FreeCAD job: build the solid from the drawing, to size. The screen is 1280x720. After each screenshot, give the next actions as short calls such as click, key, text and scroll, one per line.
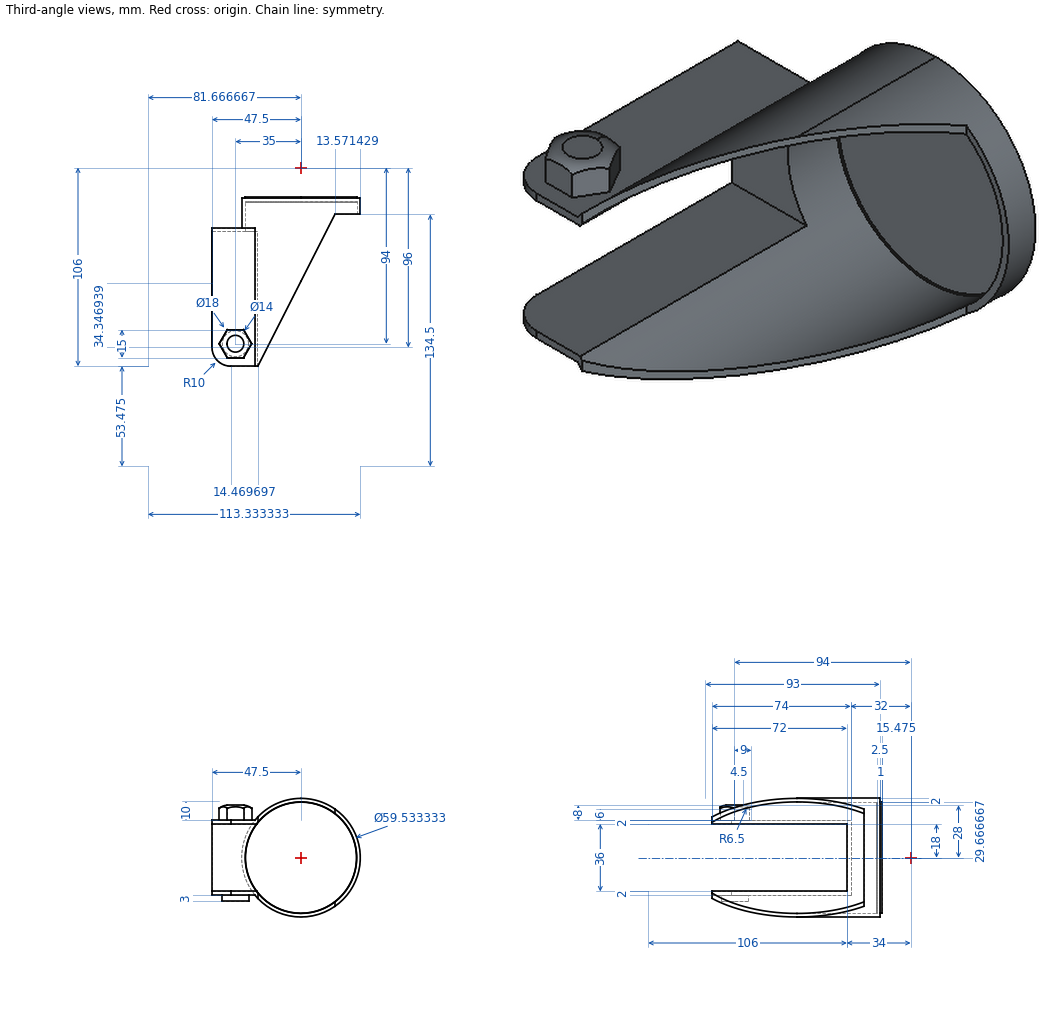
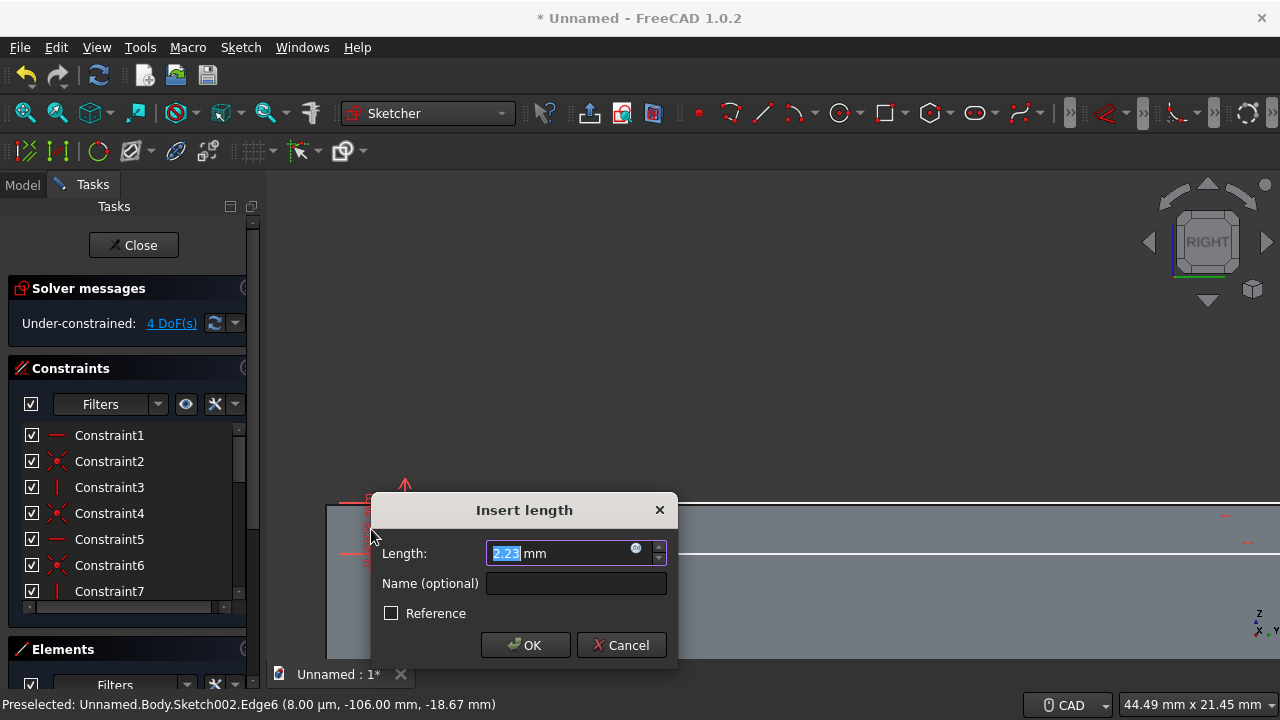
text(2)
key(Return)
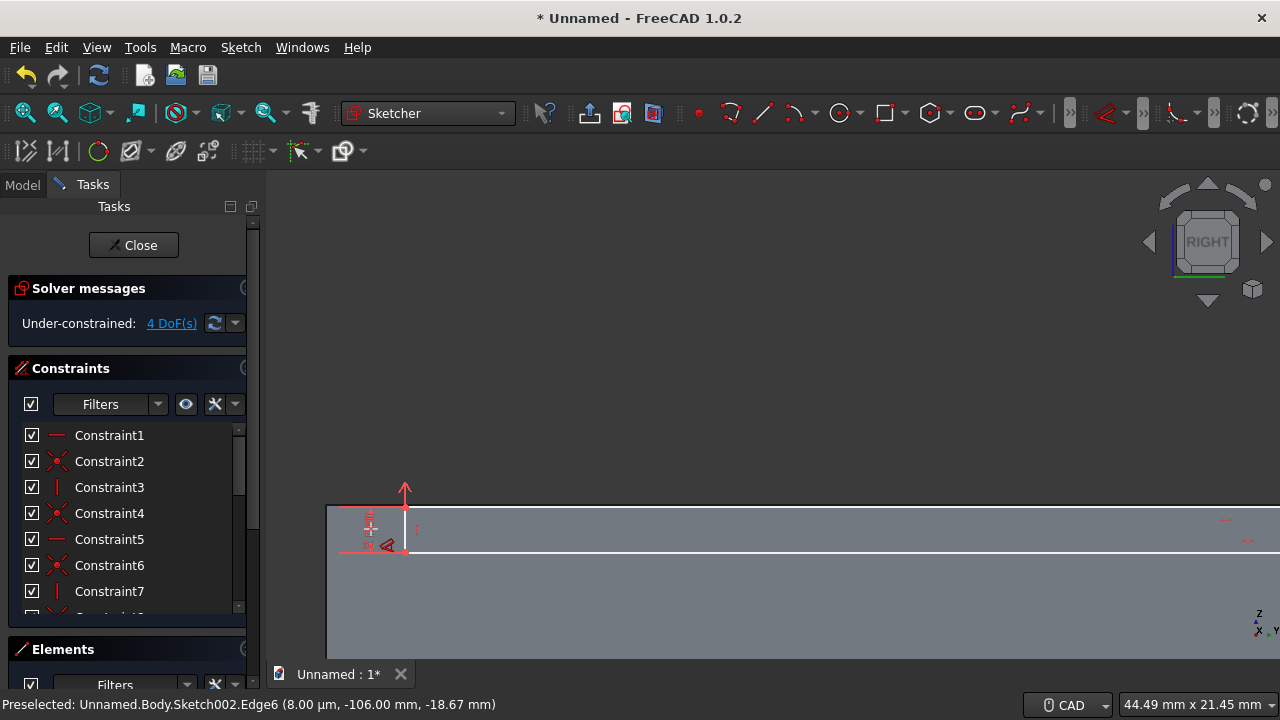
scroll(407, 519, down, 7)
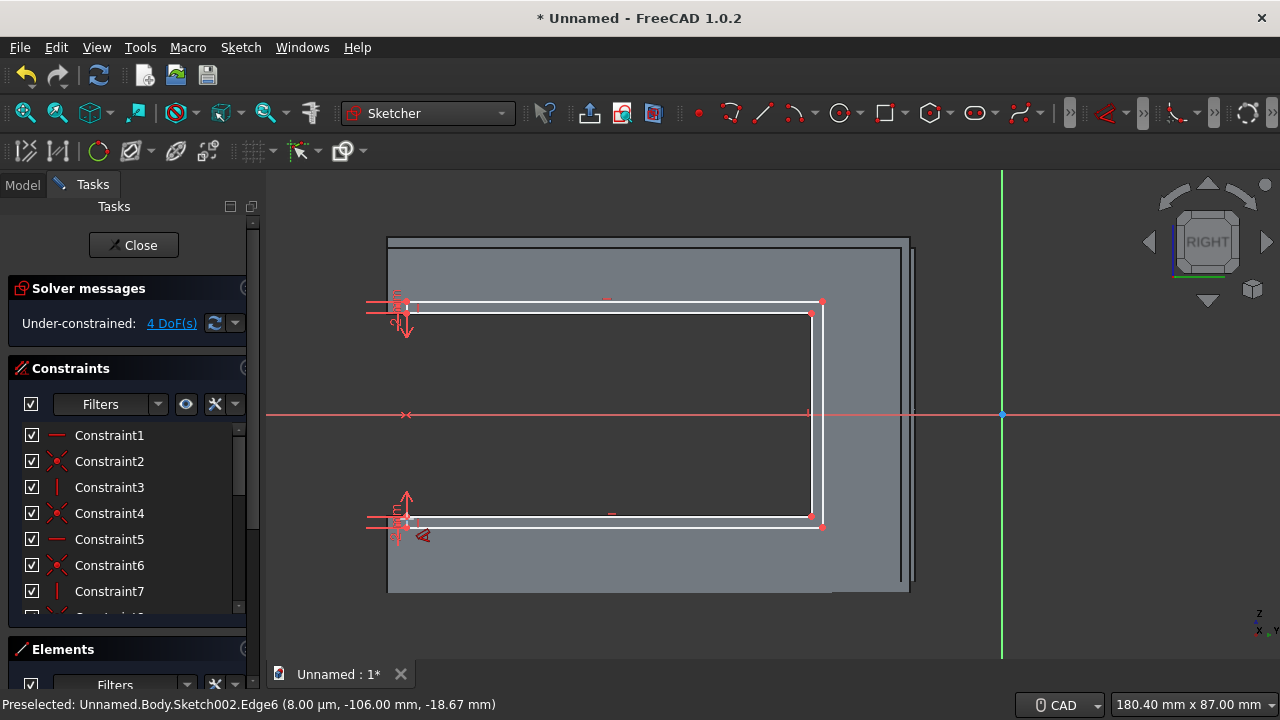
scroll(698, 302, up, 2)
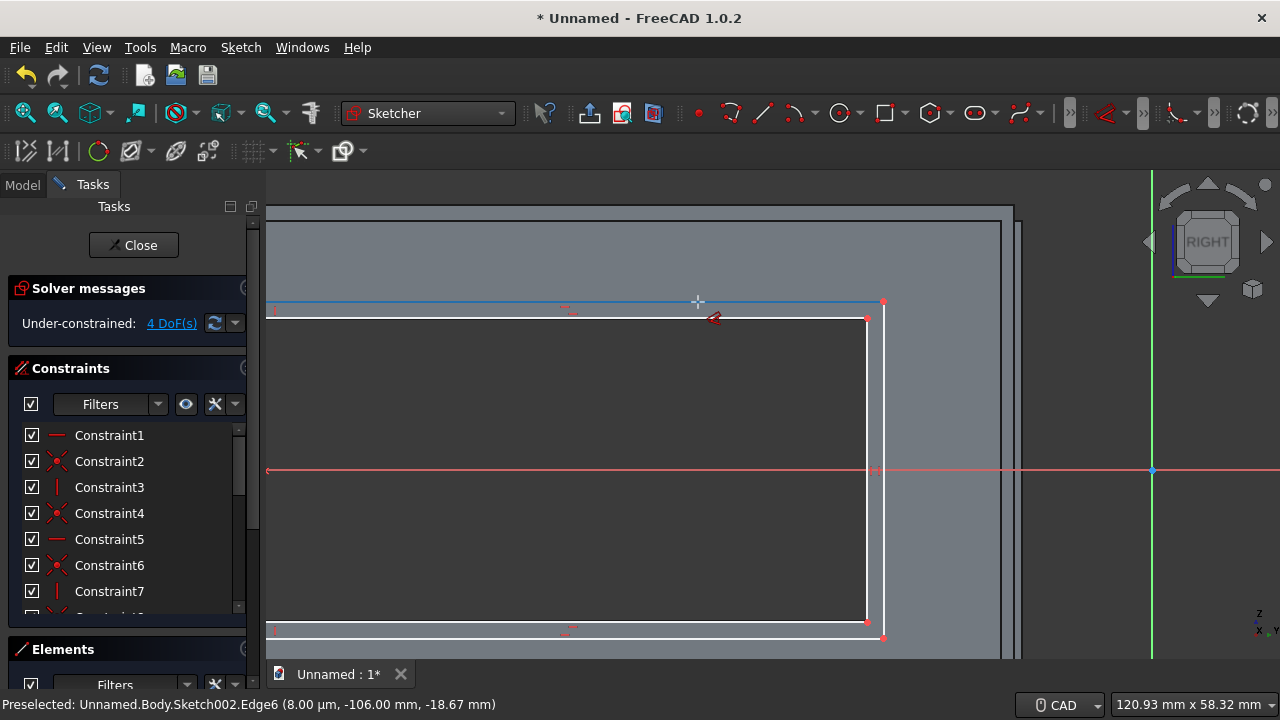
click(698, 302)
click(589, 268)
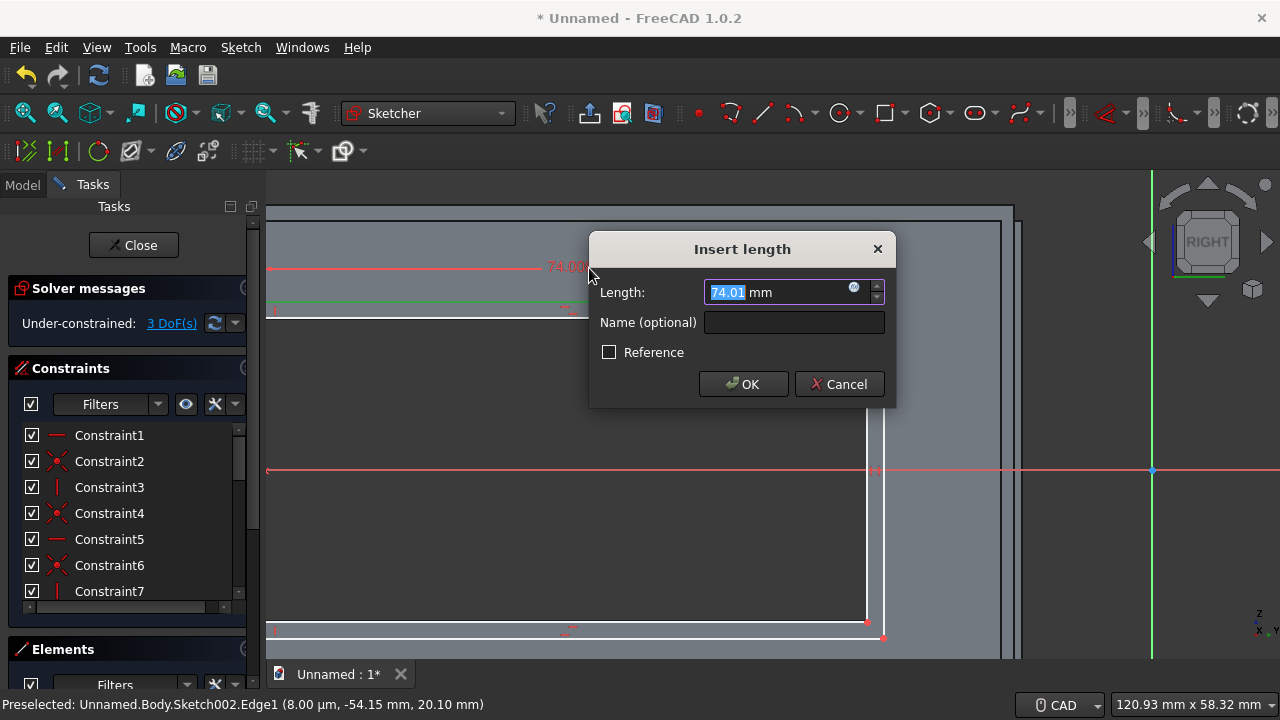
text(74)
key(Return)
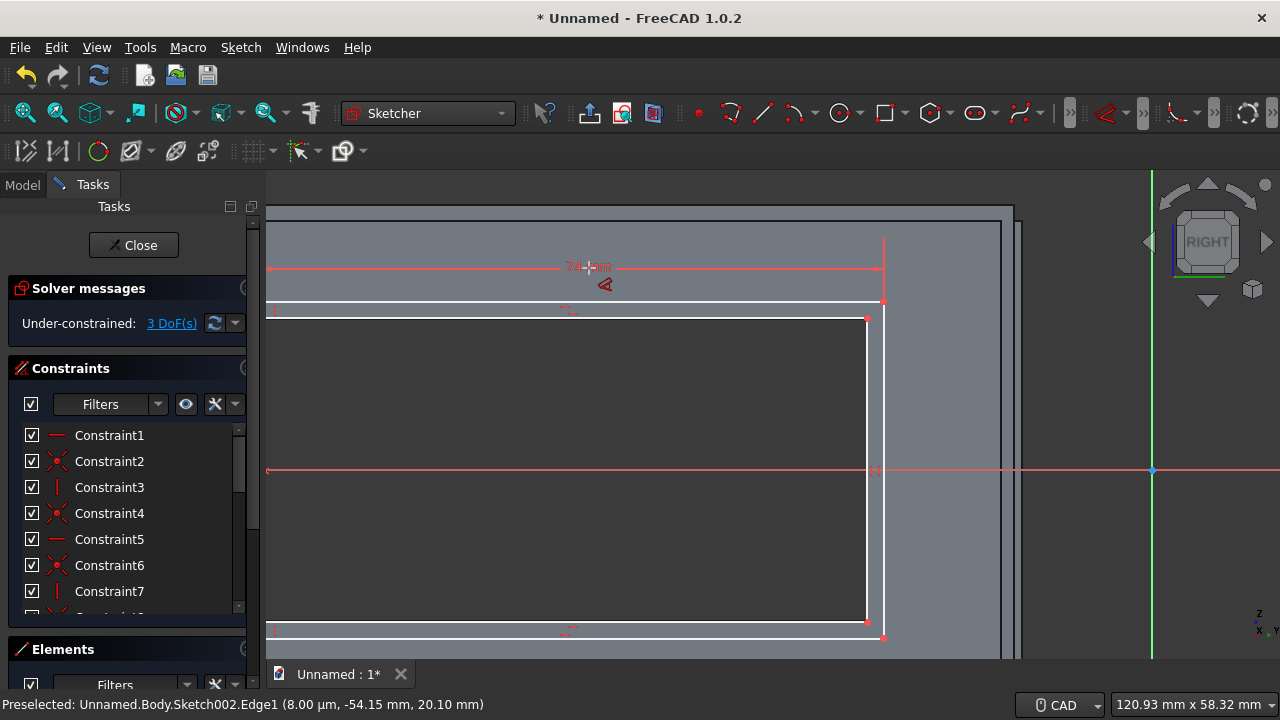
click(444, 318)
click(449, 284)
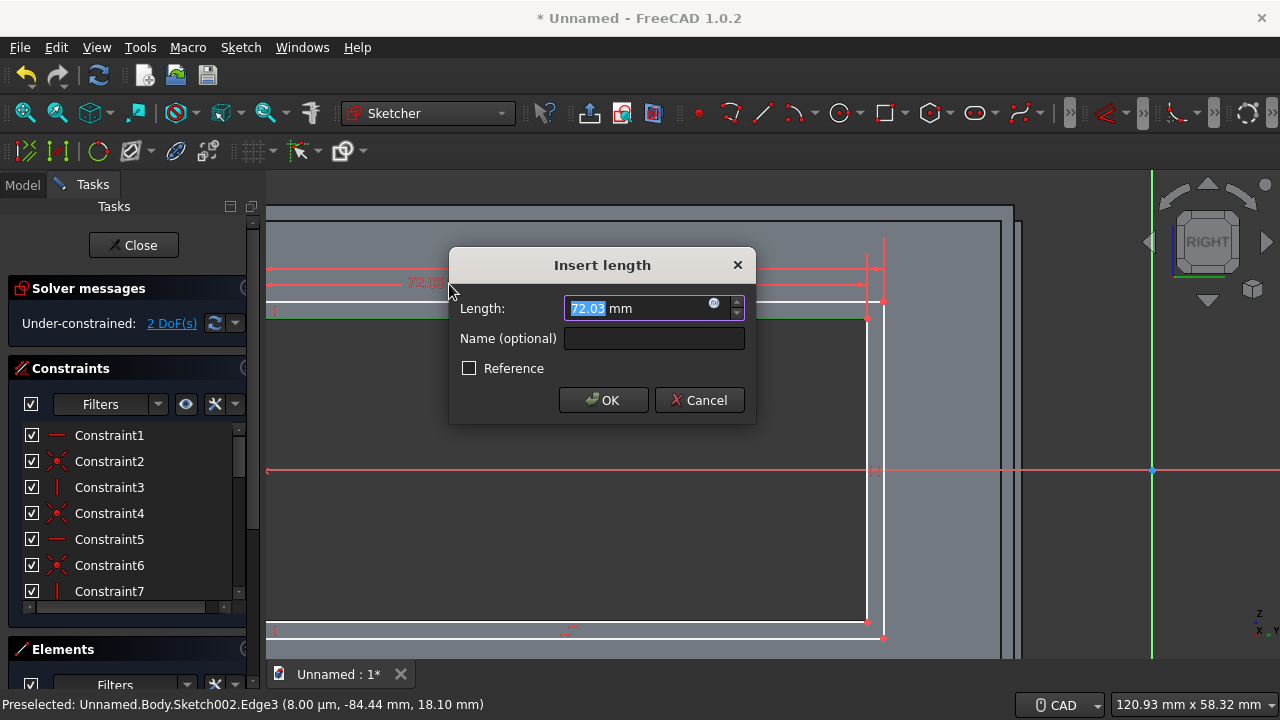
text(72)
key(Return)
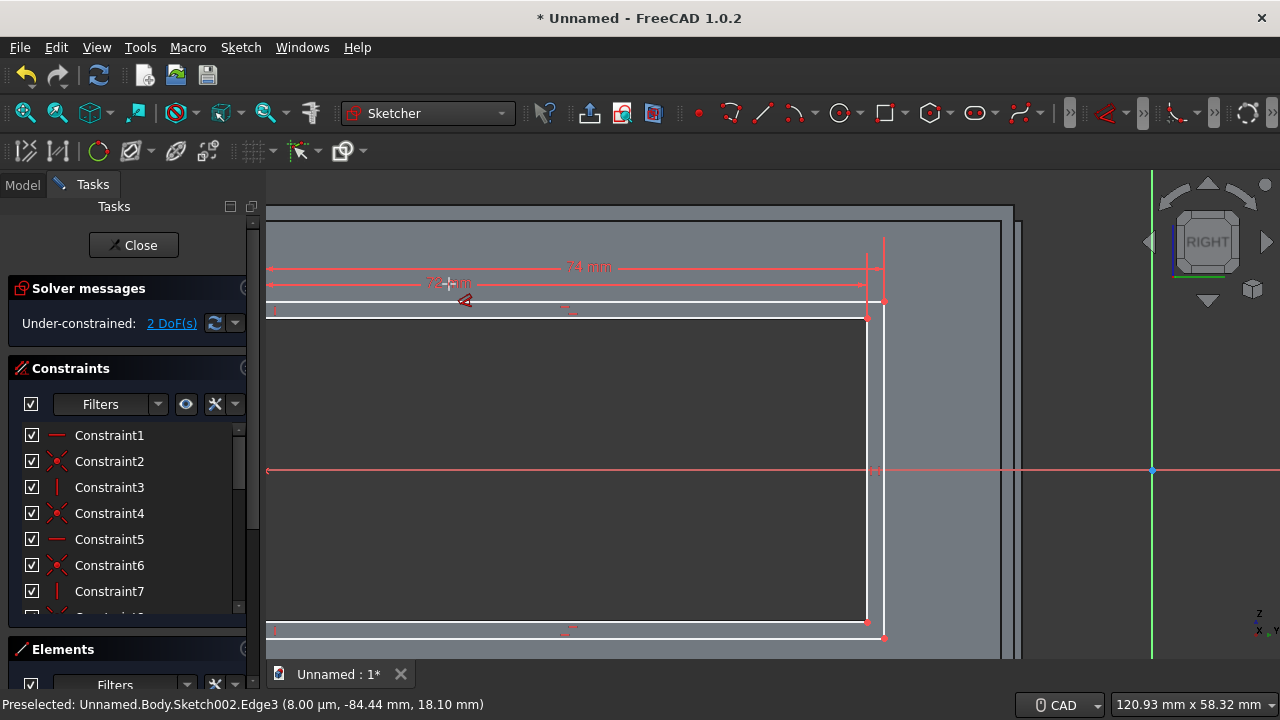
click(867, 410)
click(901, 400)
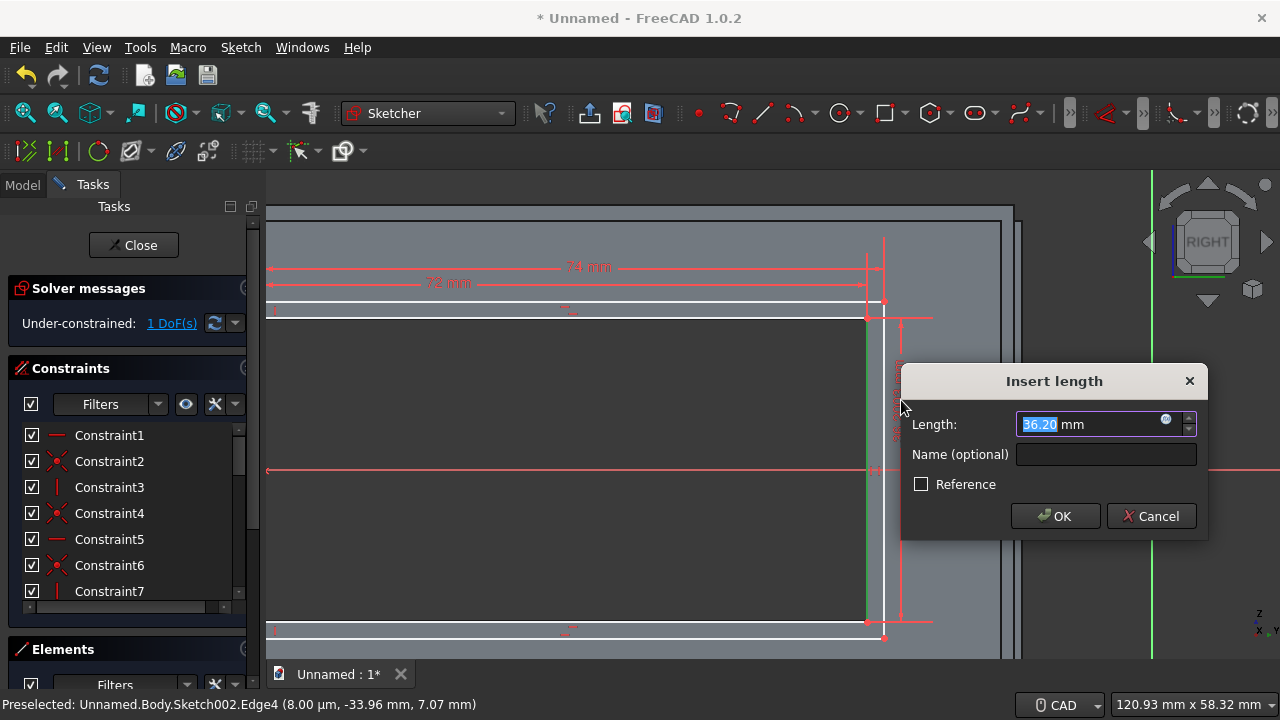
text(36)
key(Return)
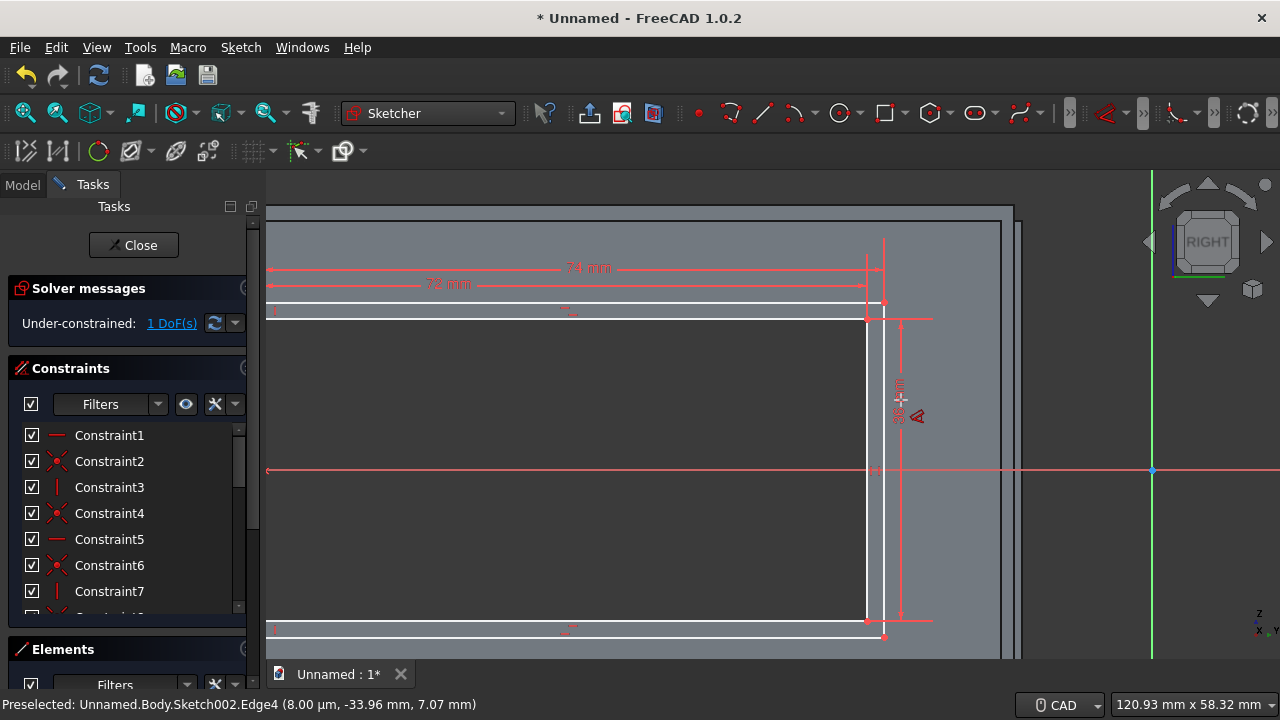
click(884, 303)
click(1000, 269)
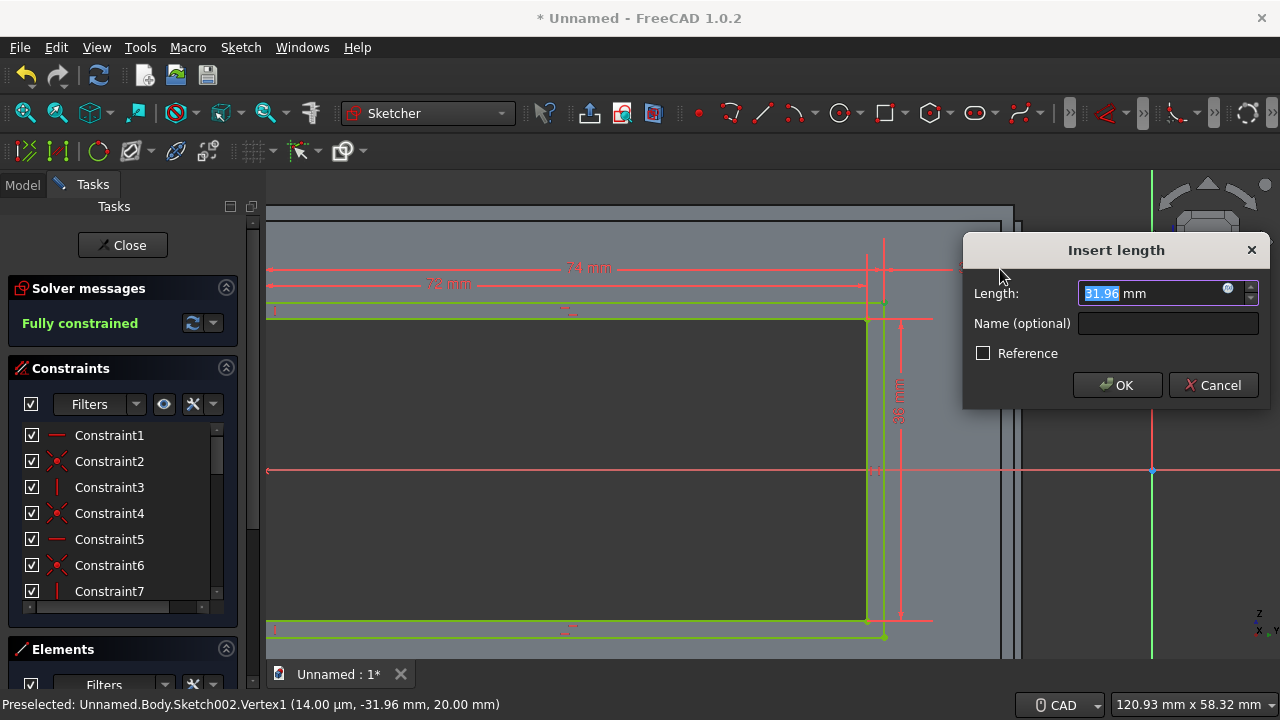
text(32)
key(Return)
key(Escape)